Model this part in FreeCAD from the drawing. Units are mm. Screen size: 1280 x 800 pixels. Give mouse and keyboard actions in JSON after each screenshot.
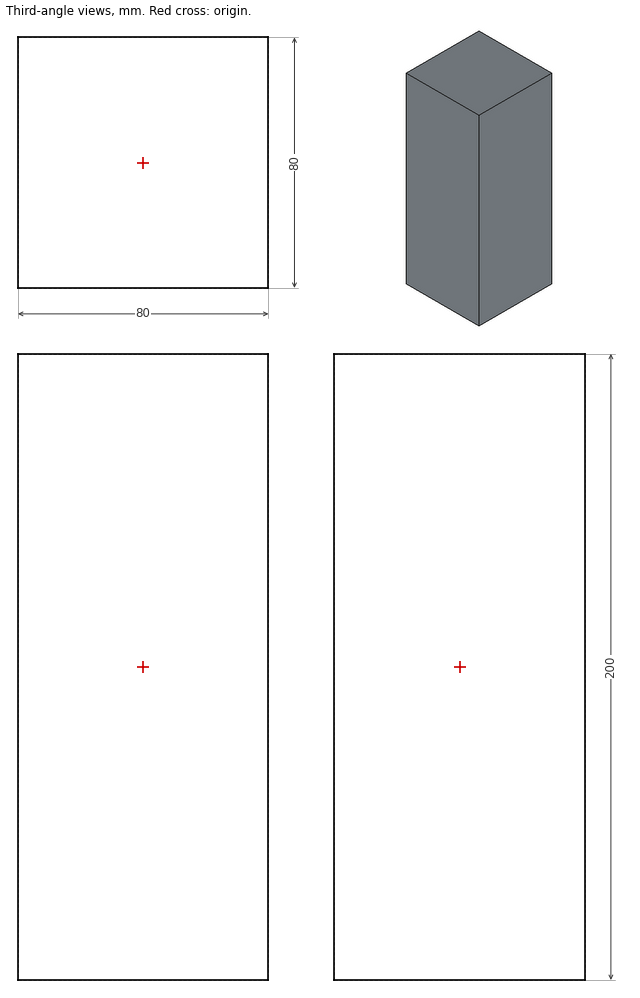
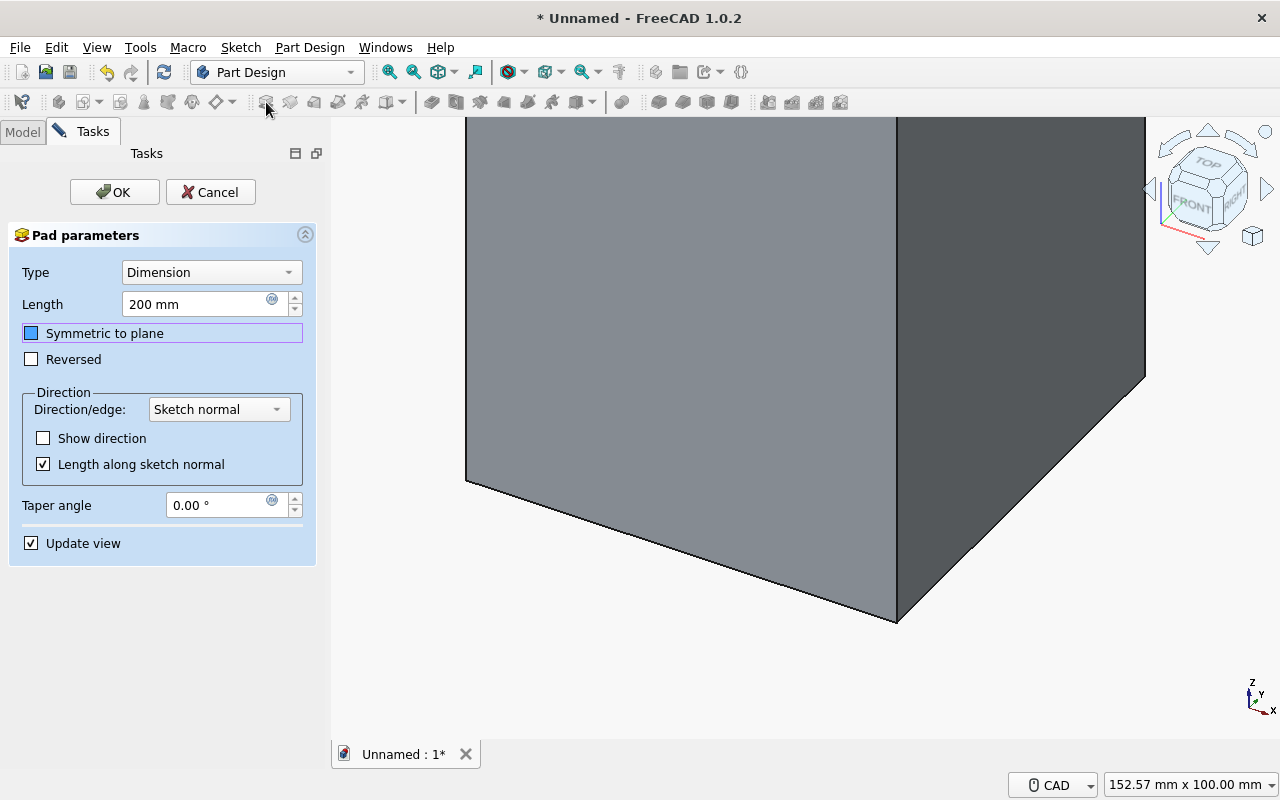
{"action": "left_click", "coordinate": [30, 333]}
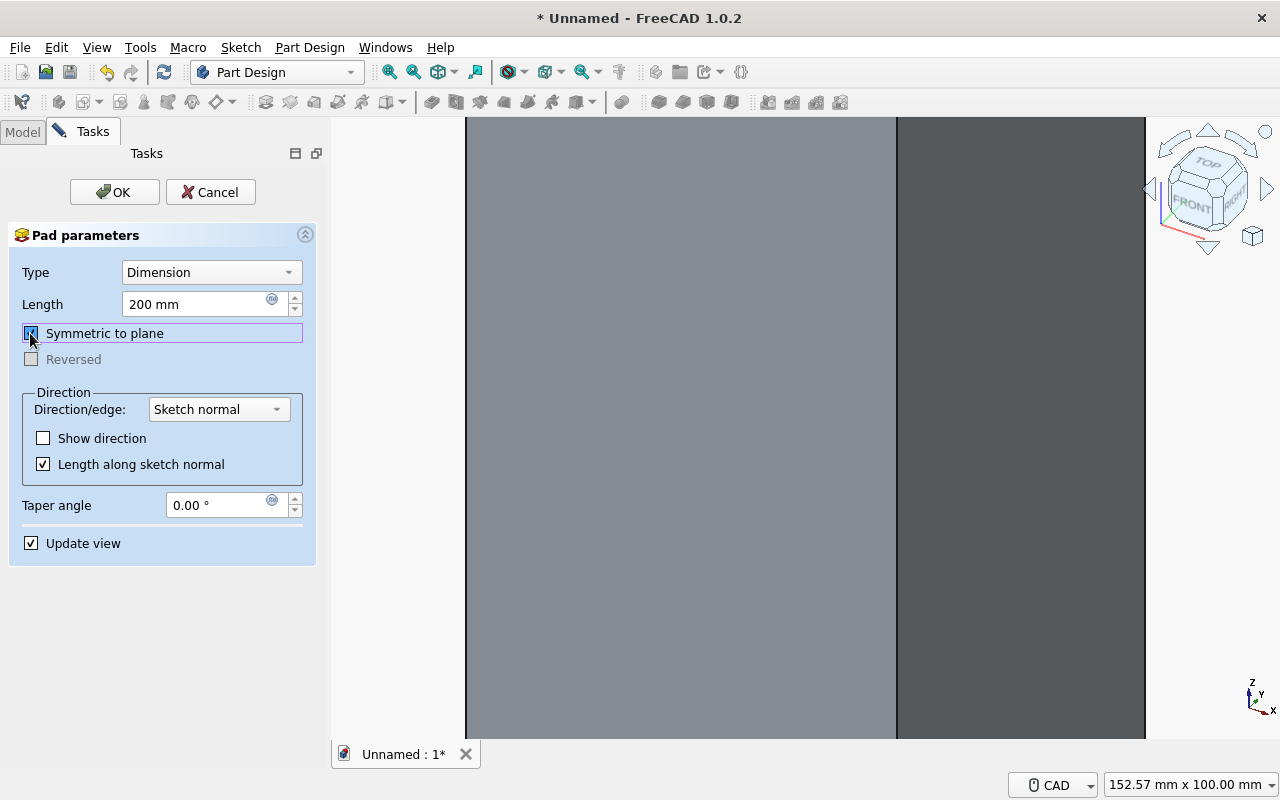
{"action": "left_click", "coordinate": [115, 192]}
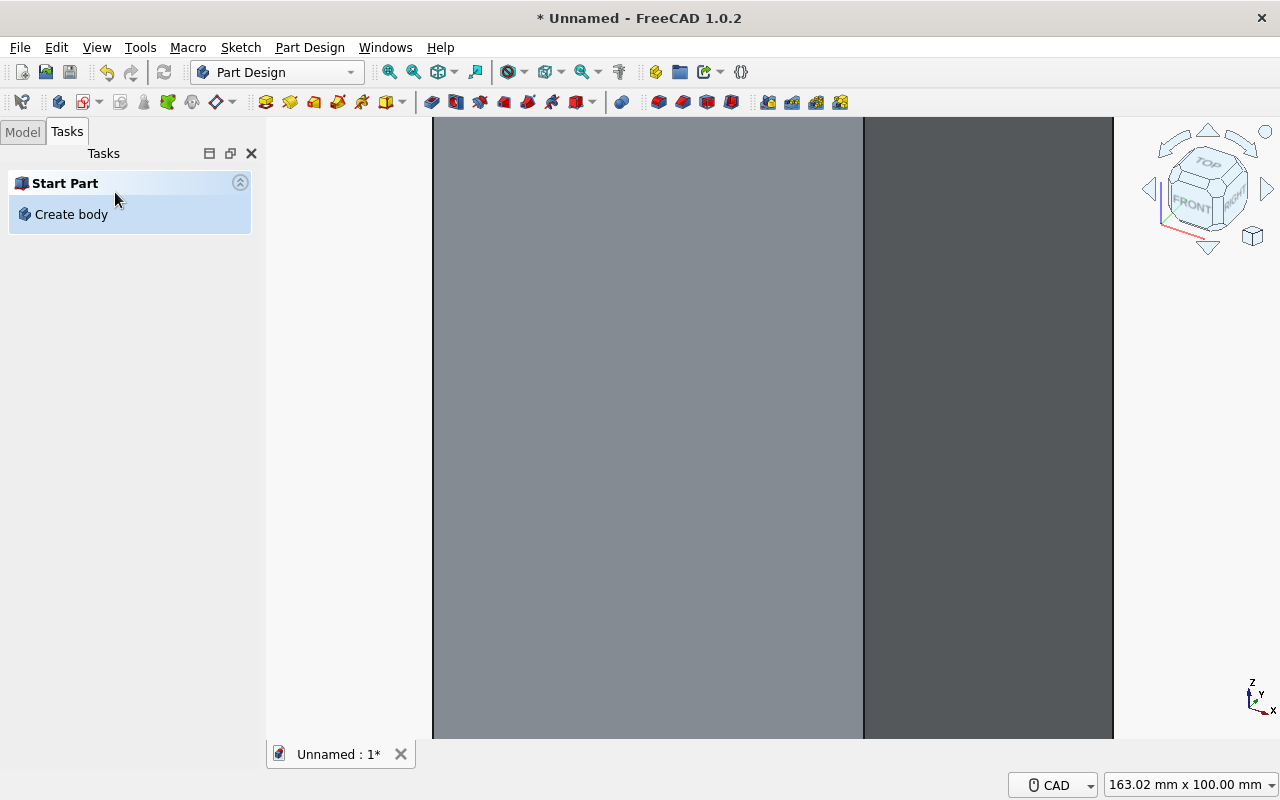
{"action": "key", "text": "0"}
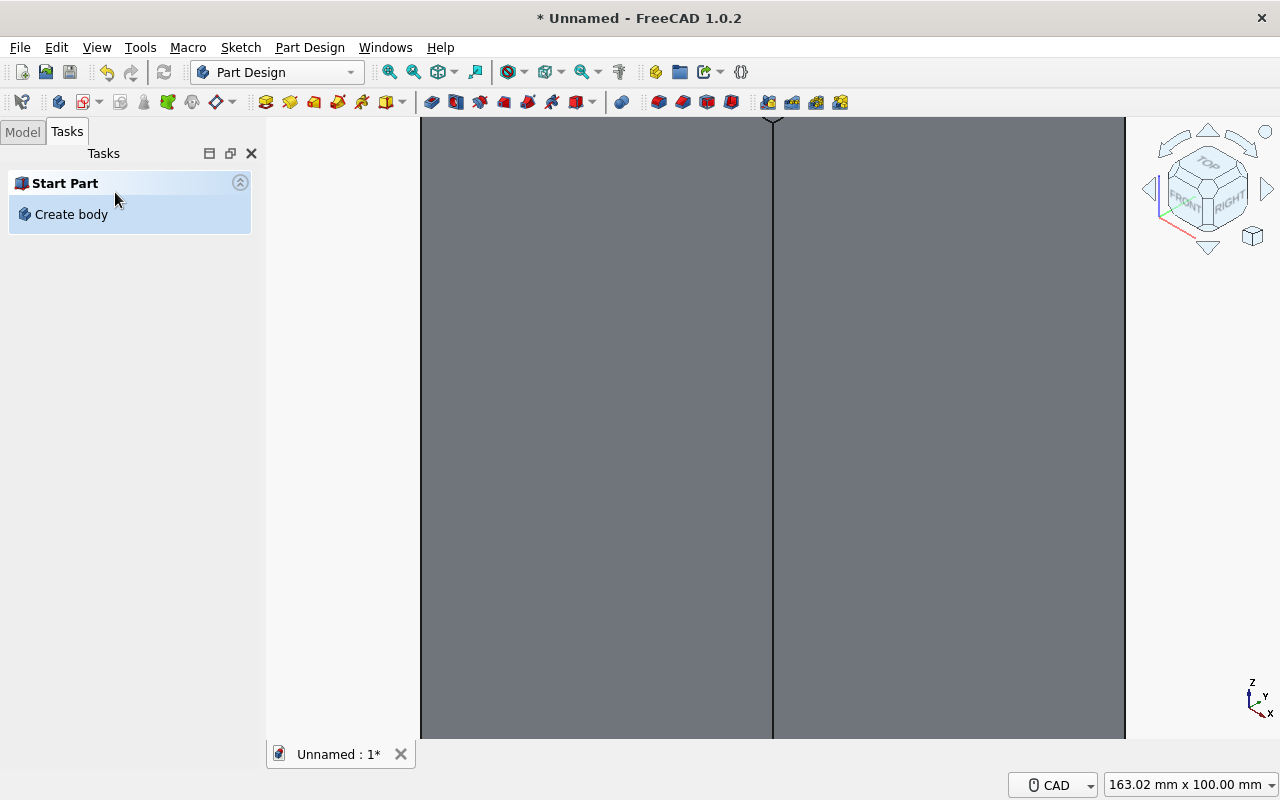
{"action": "left_click", "coordinate": [390, 72]}